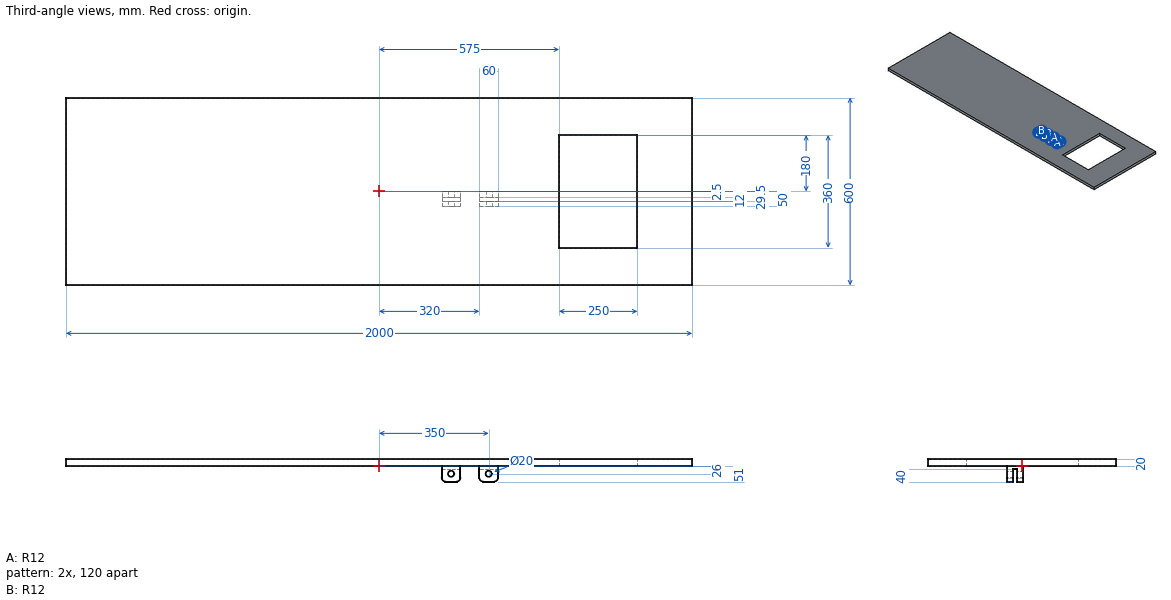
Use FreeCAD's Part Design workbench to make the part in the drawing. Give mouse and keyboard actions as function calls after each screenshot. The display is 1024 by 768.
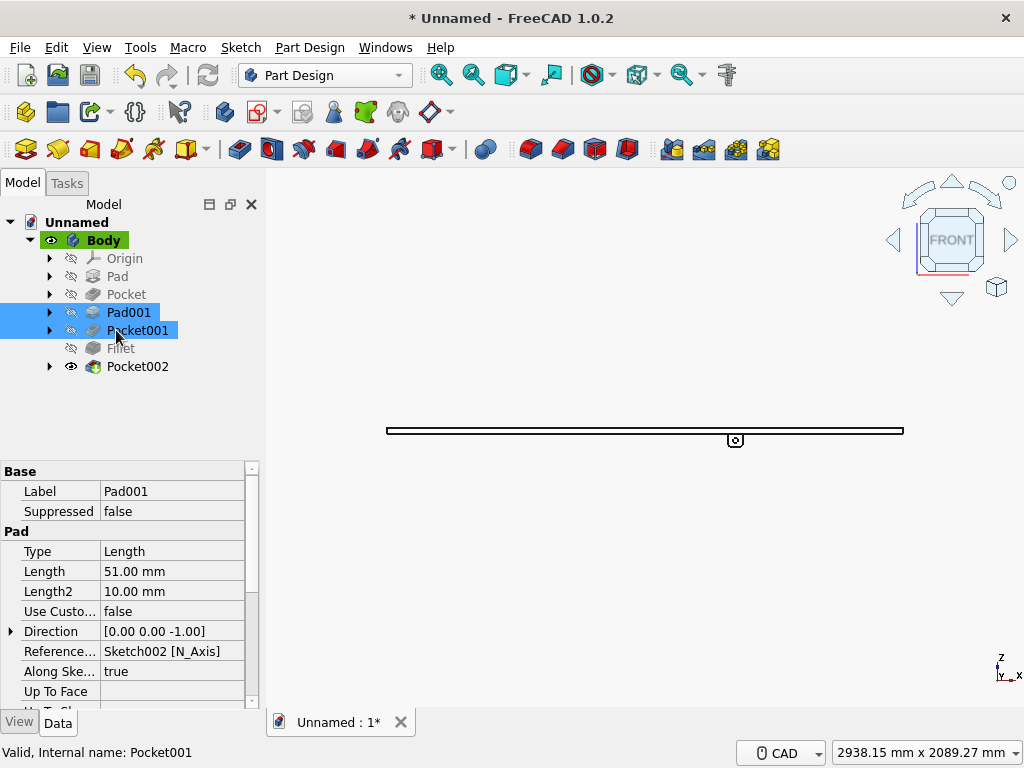
click(116, 366, ctrl)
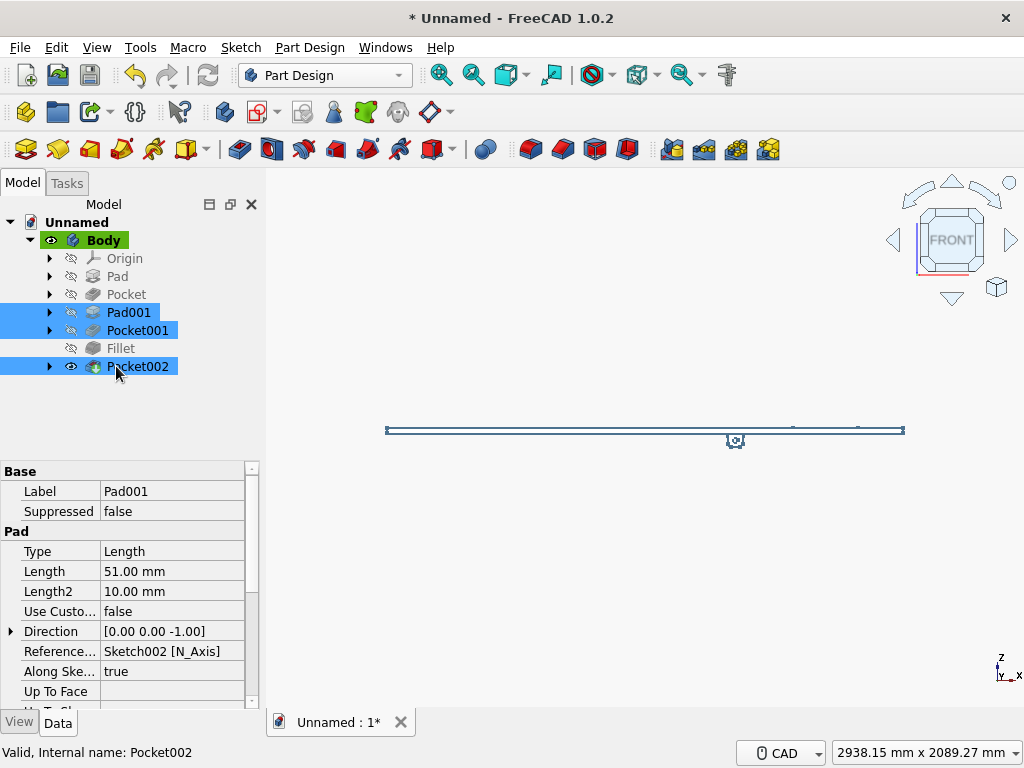
click(704, 150)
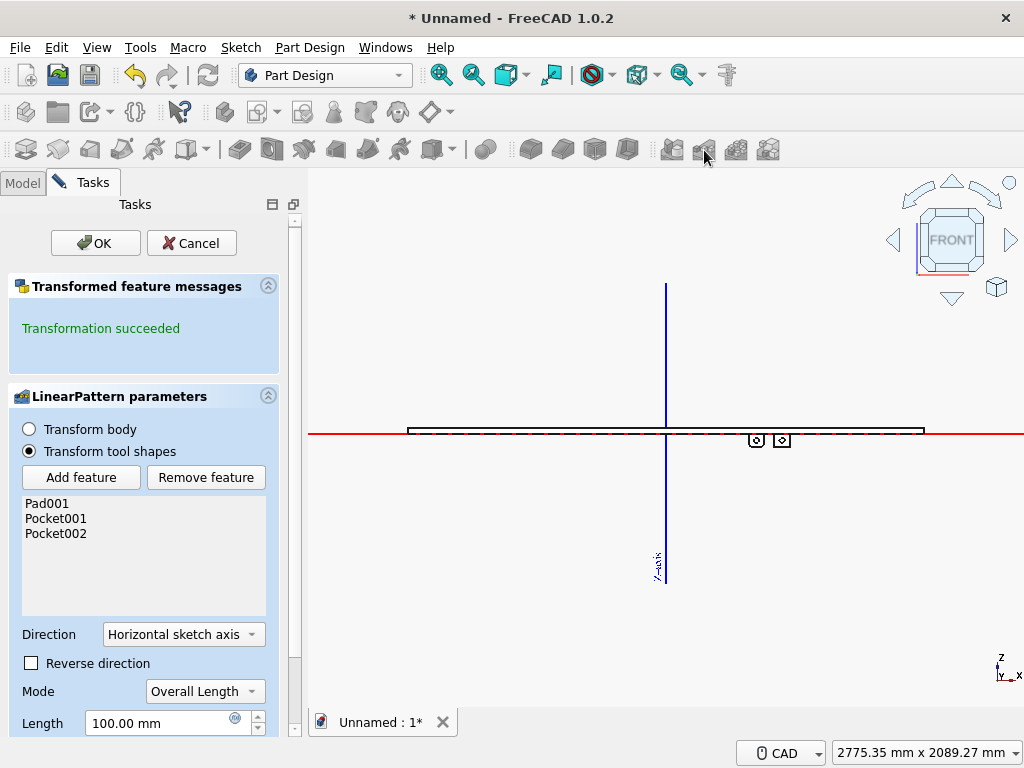
click(184, 634)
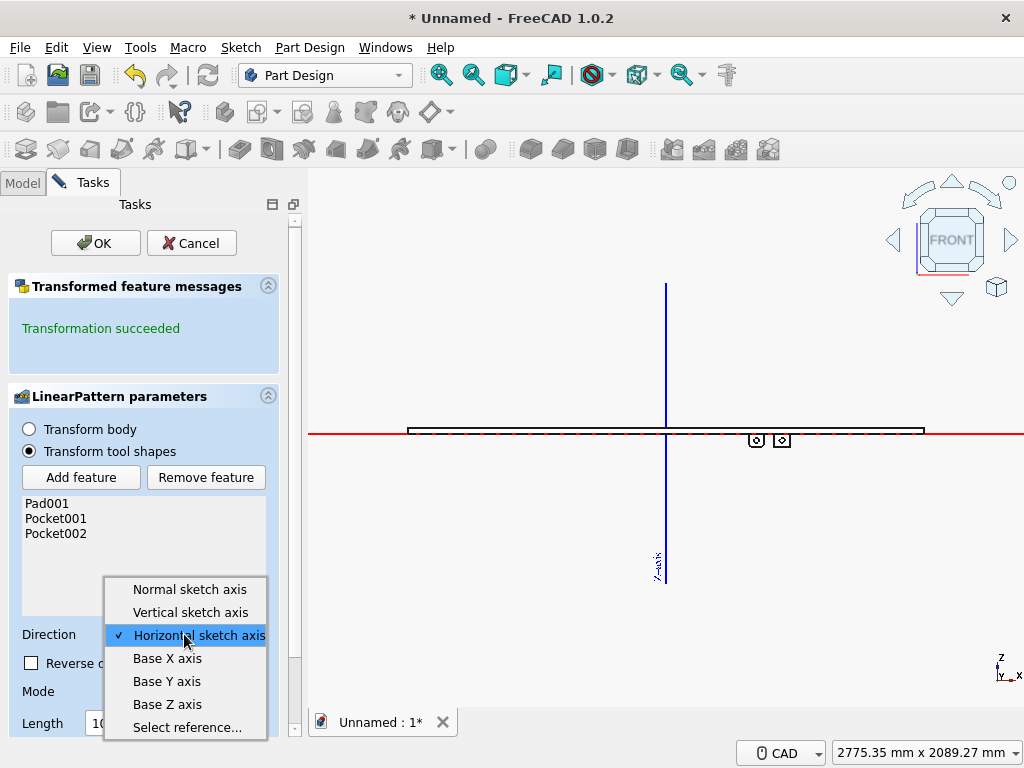
click(184, 658)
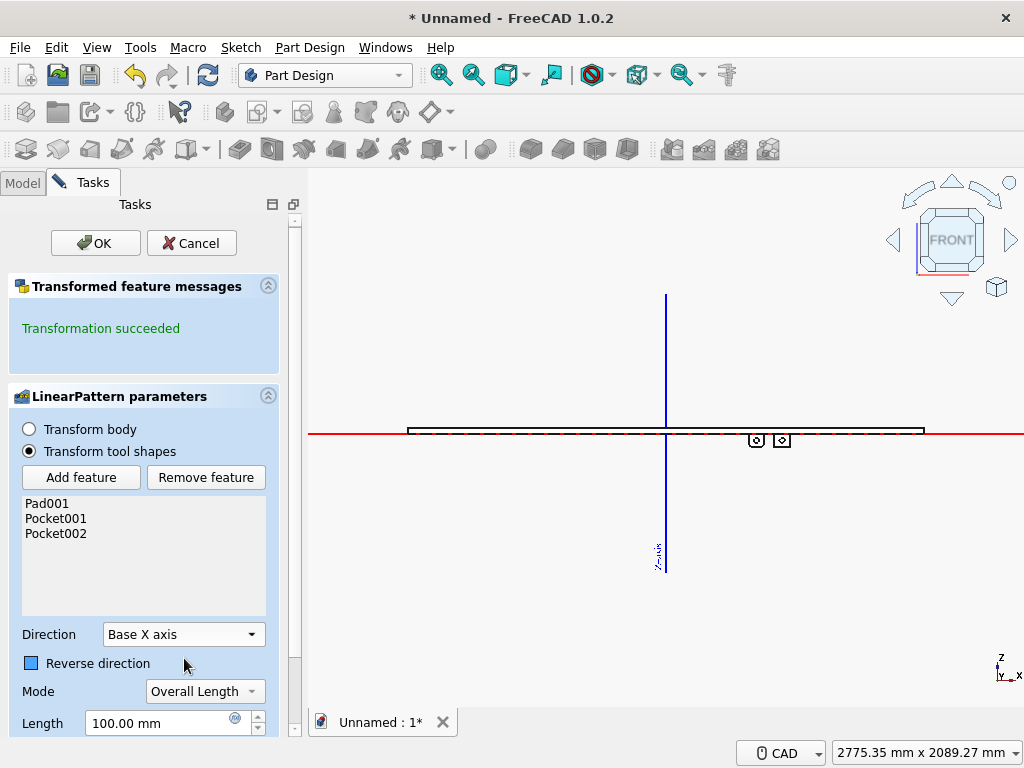
click(206, 692)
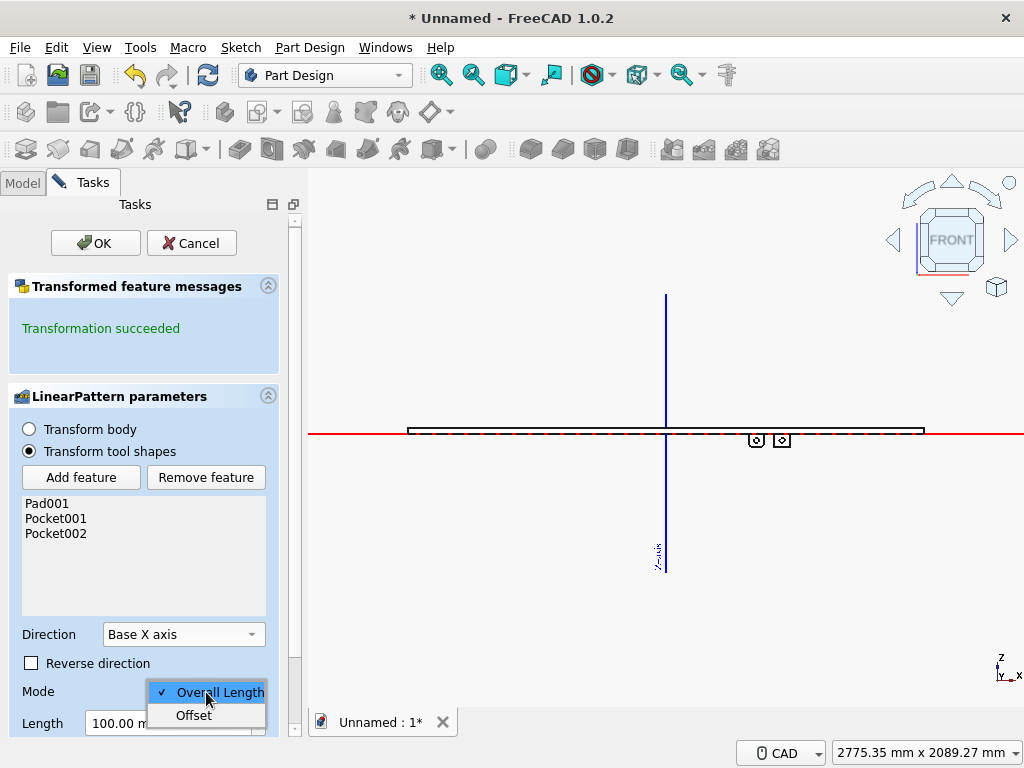
click(206, 716)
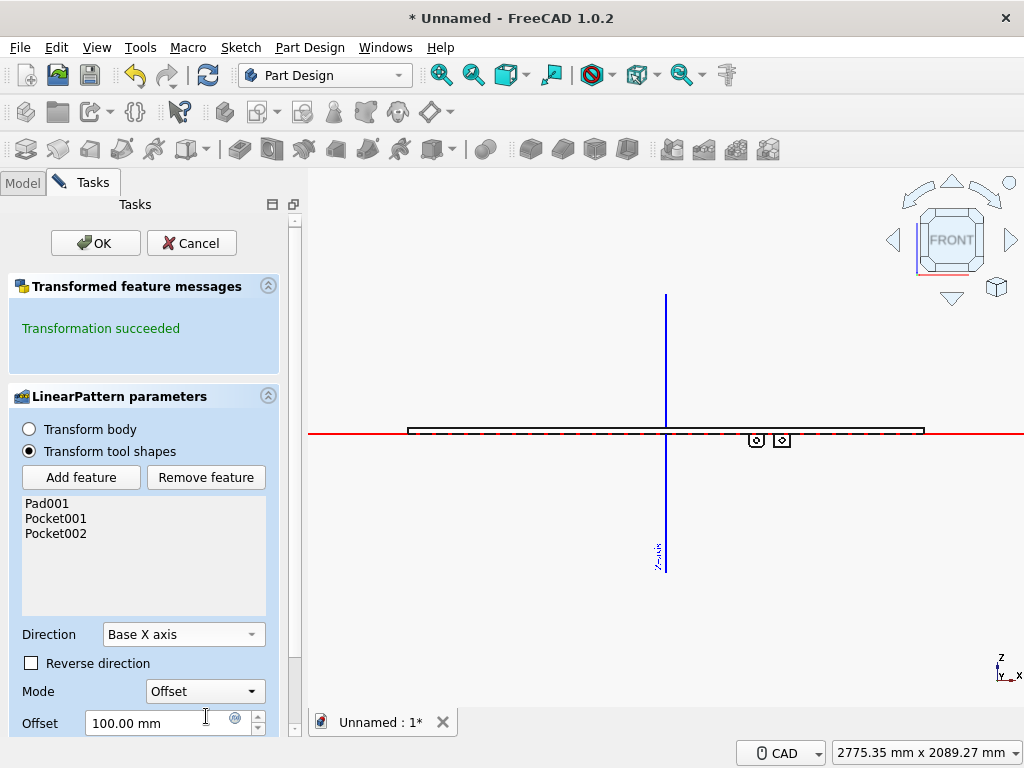
triple_click(168, 723)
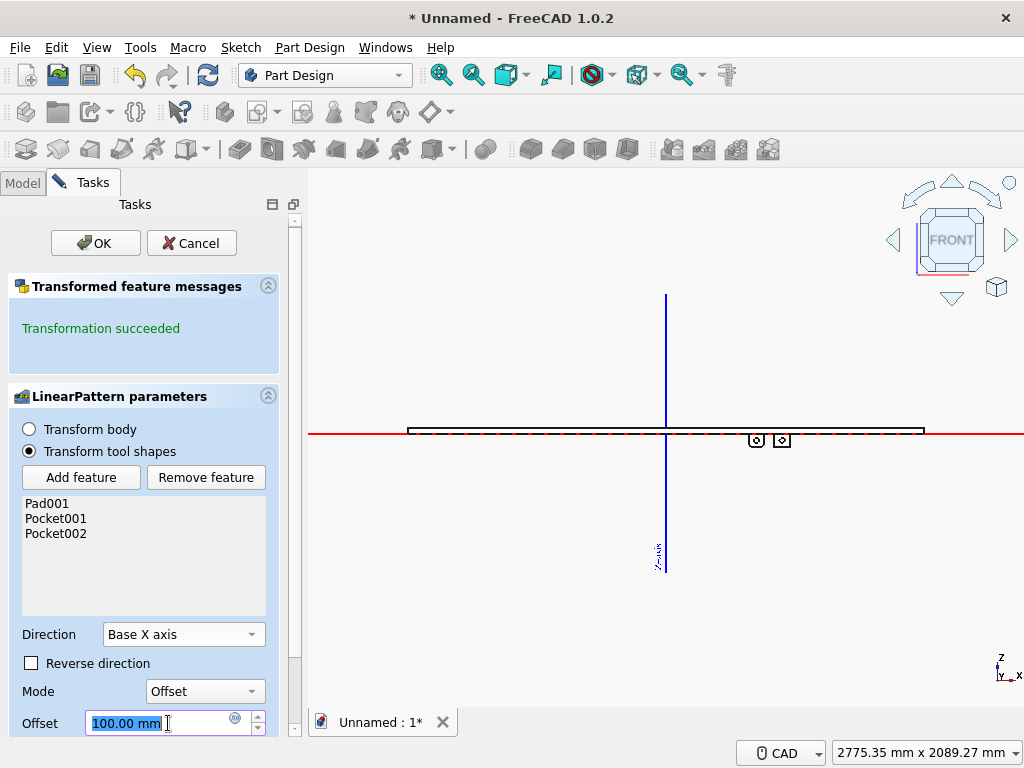
text(120)
key(Tab)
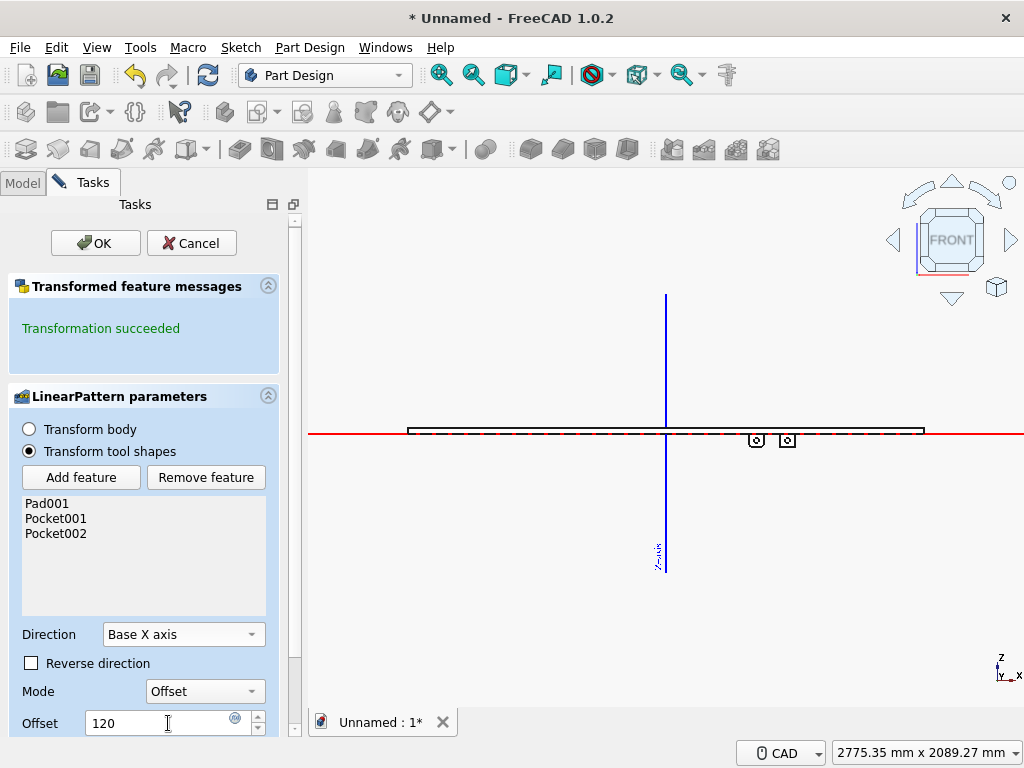
scroll(295, 475, down, 2)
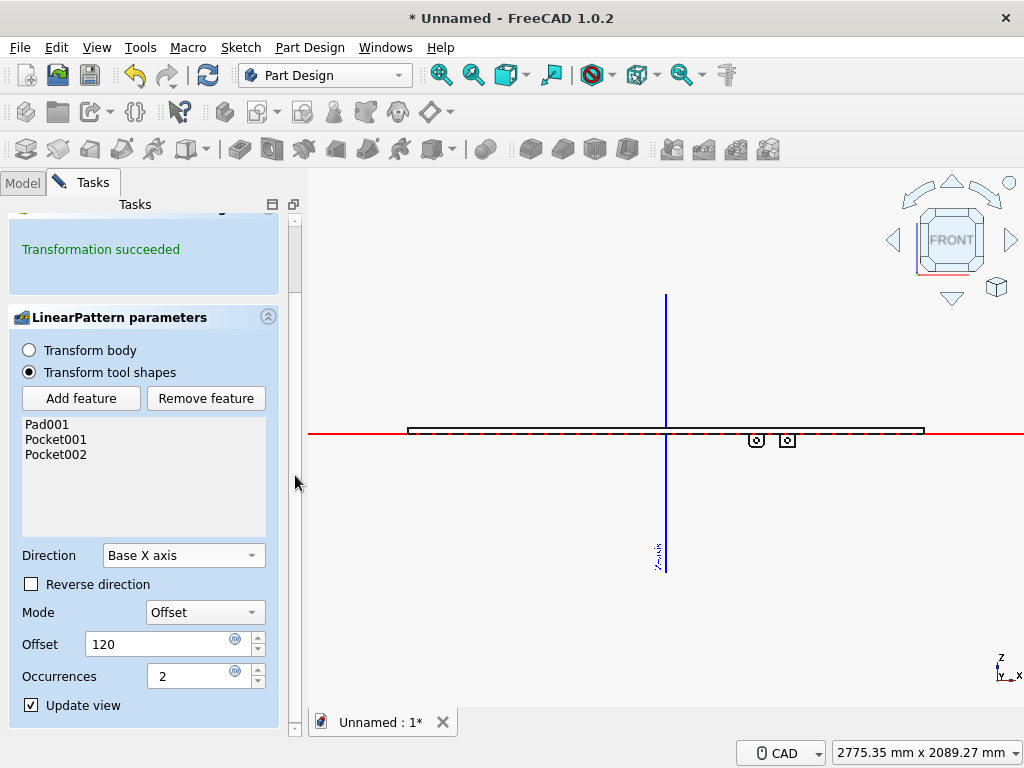
triple_click(198, 676)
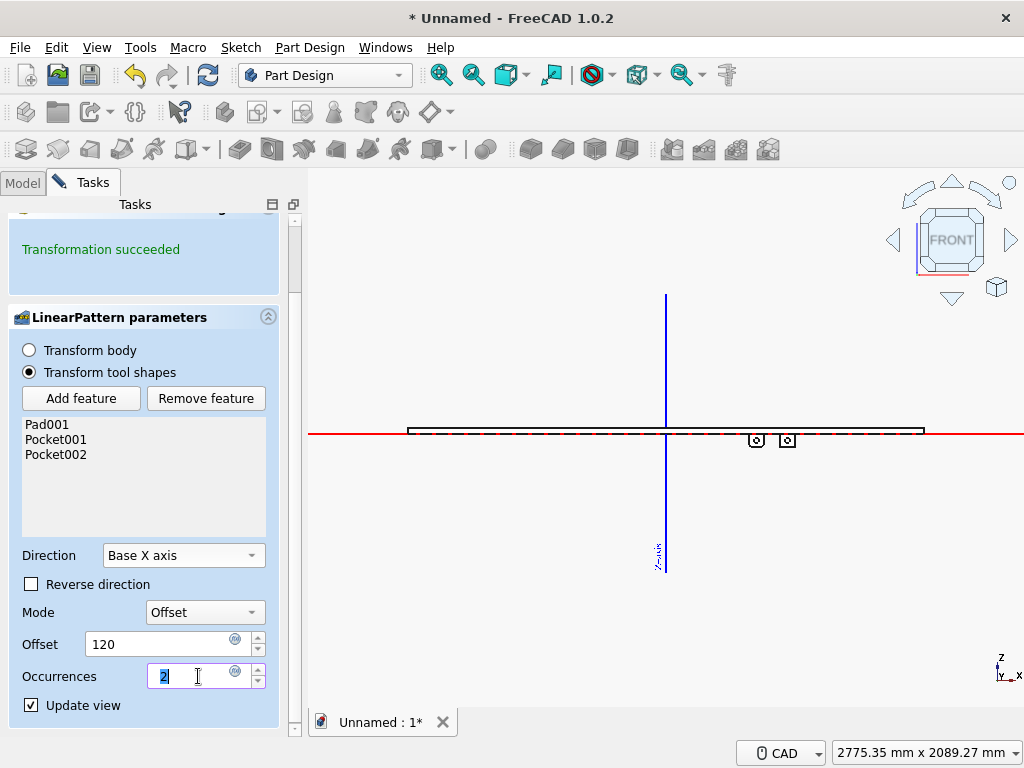
text(2)
key(Tab)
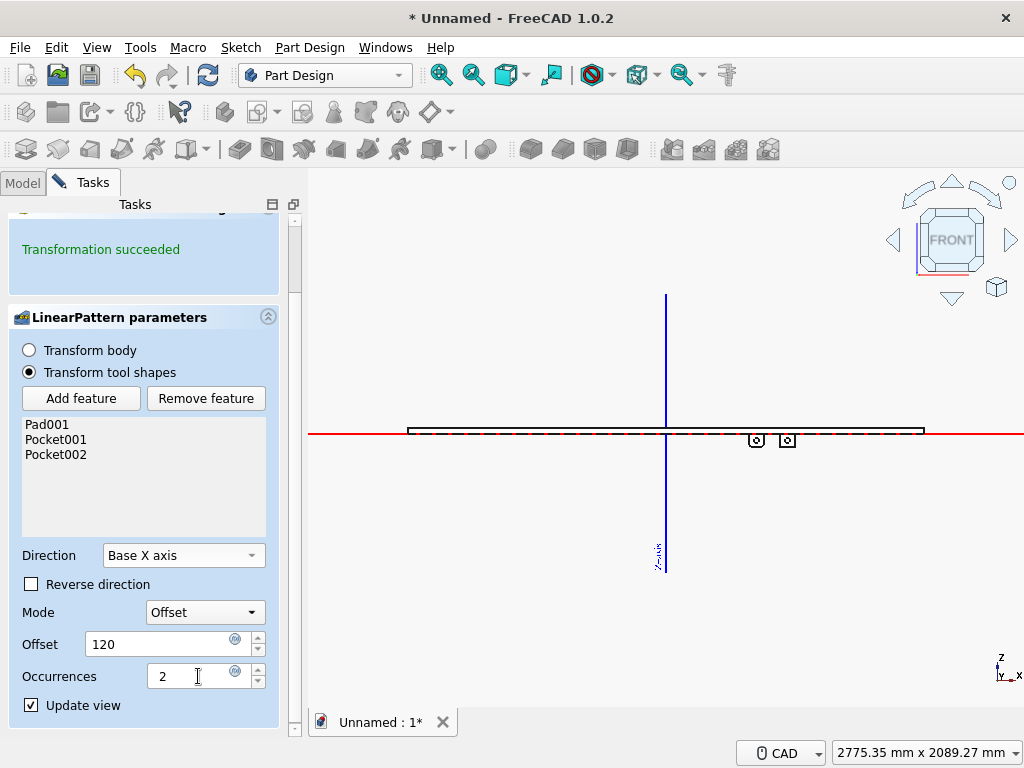
click(30, 584)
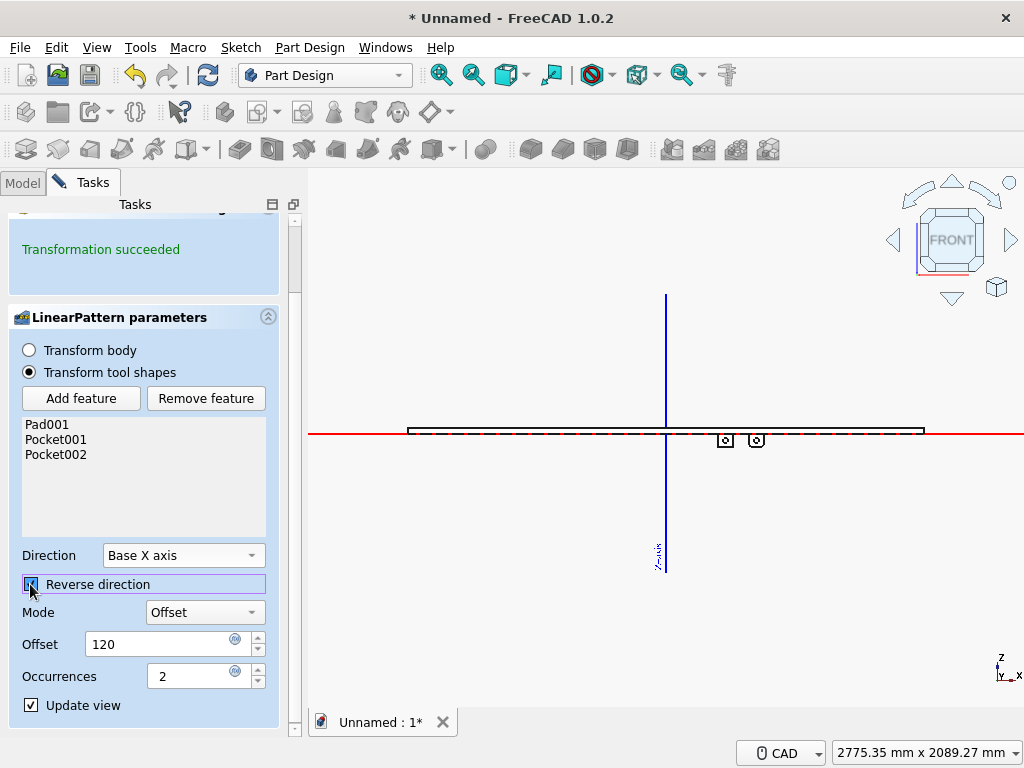
scroll(295, 475, up, 3)